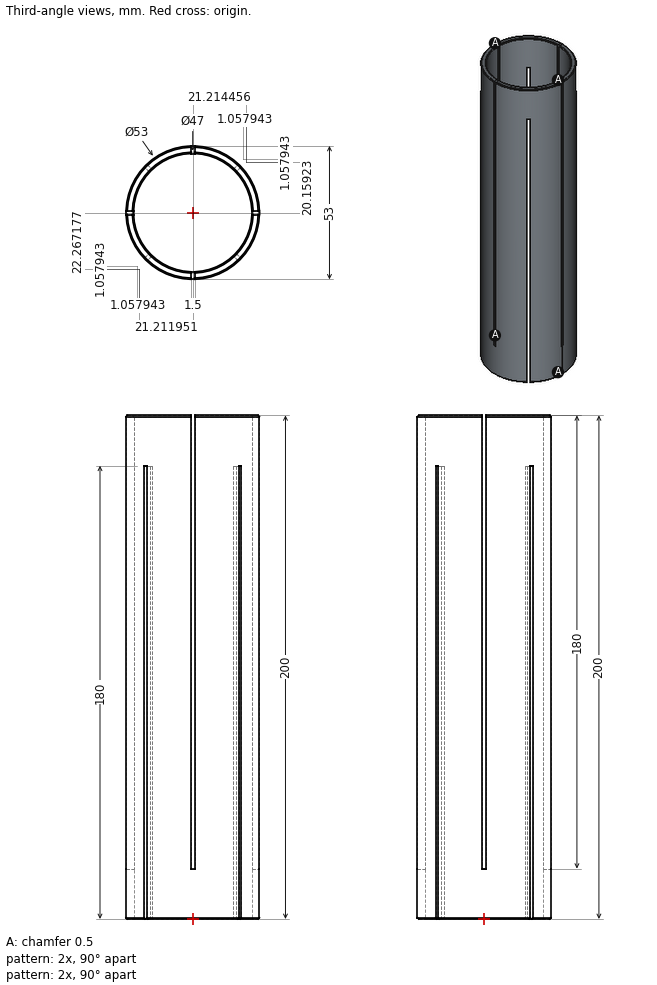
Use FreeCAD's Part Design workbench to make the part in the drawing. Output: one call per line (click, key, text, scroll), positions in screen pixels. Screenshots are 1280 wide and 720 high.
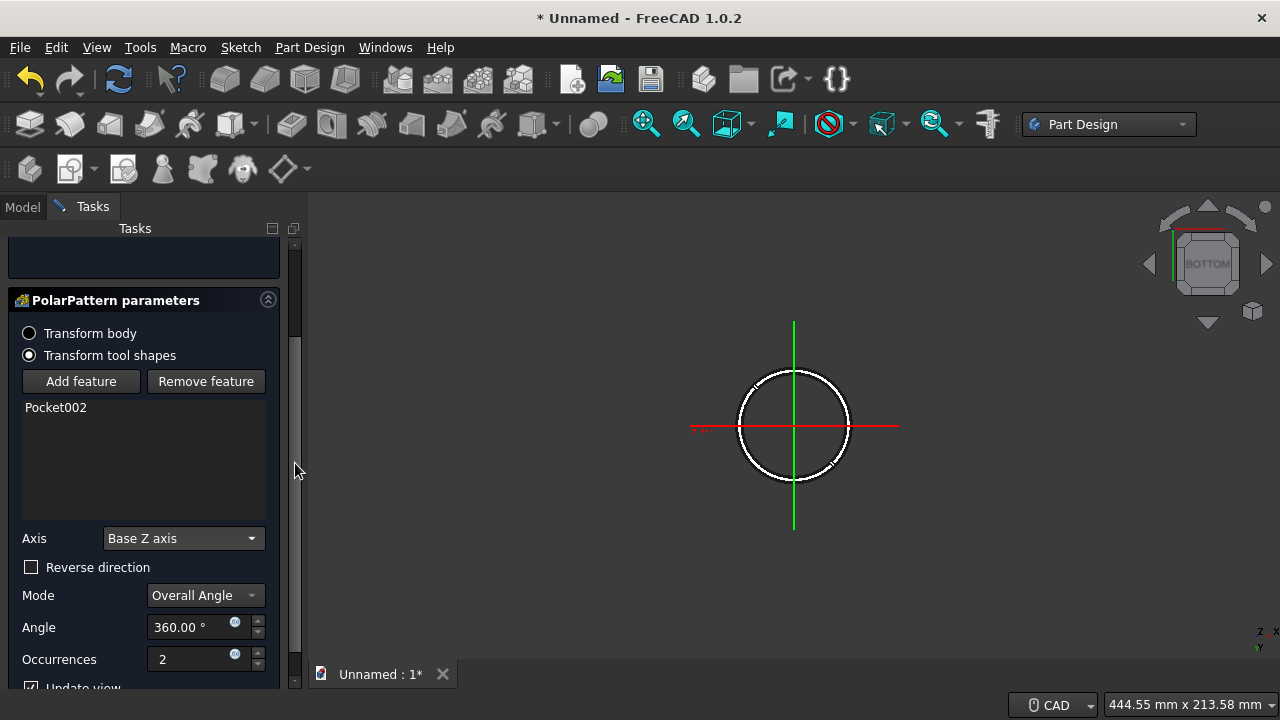
click(206, 596)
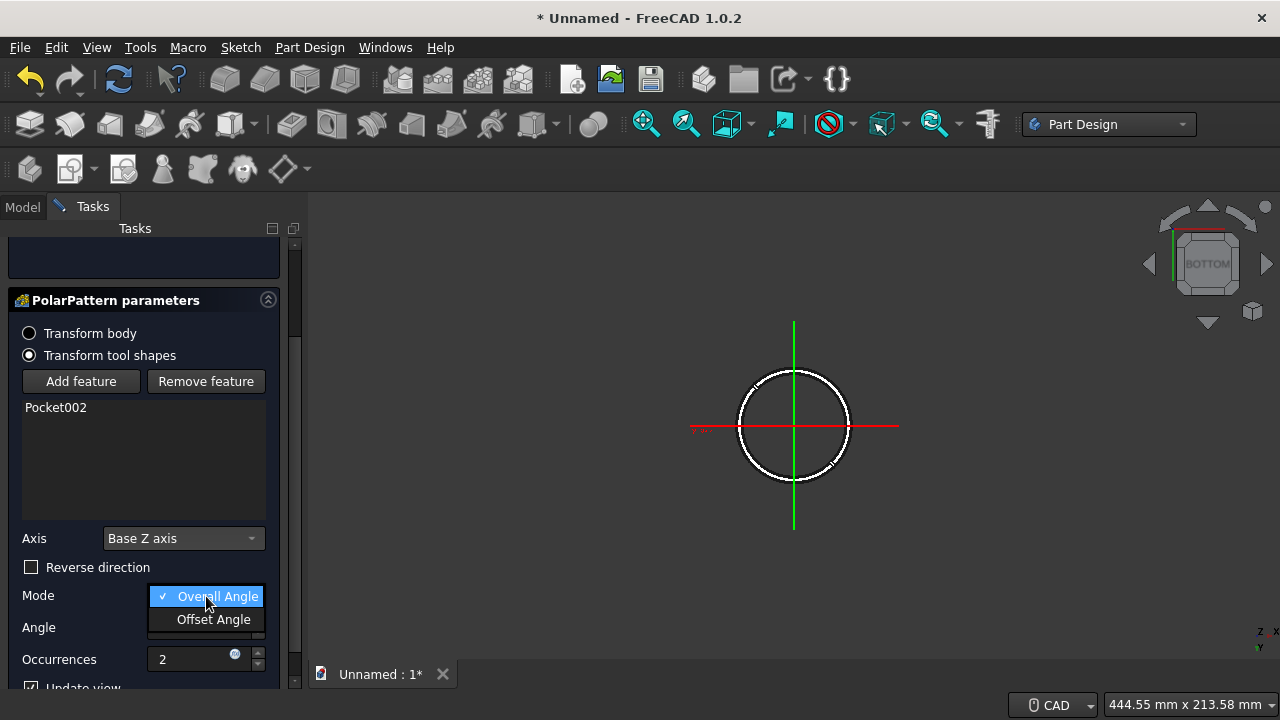
click(206, 620)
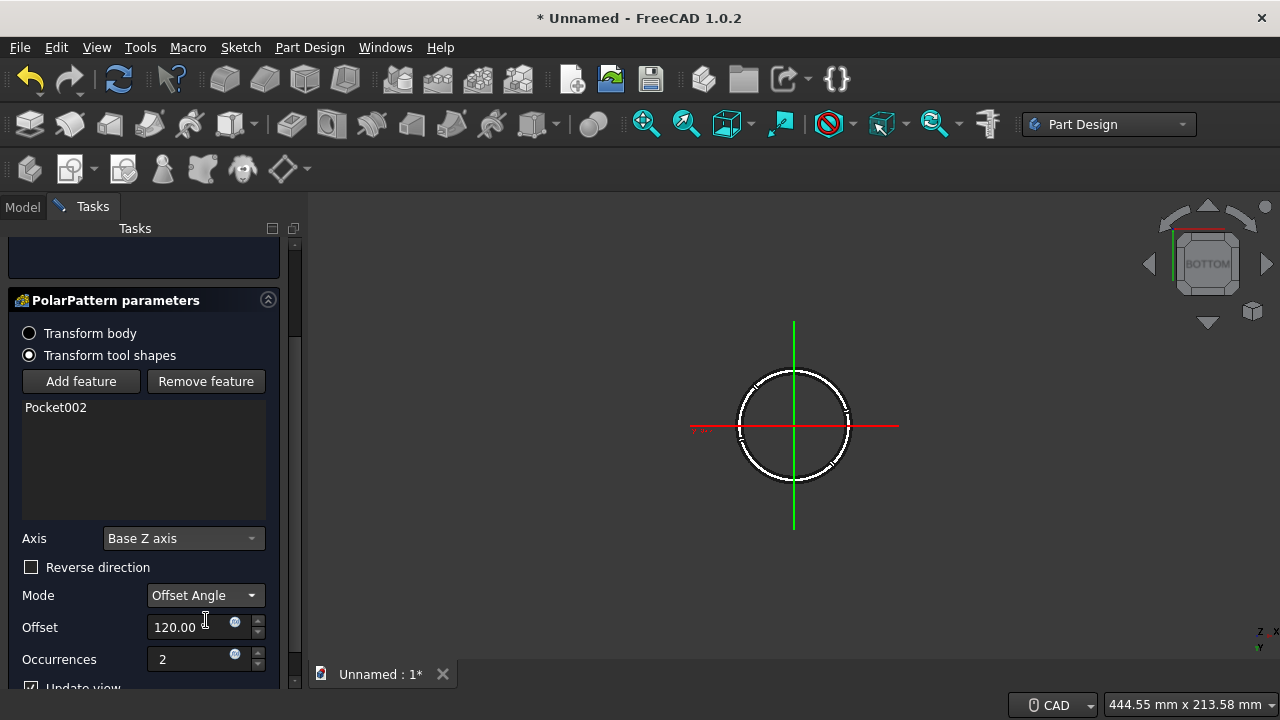
triple_click(198, 627)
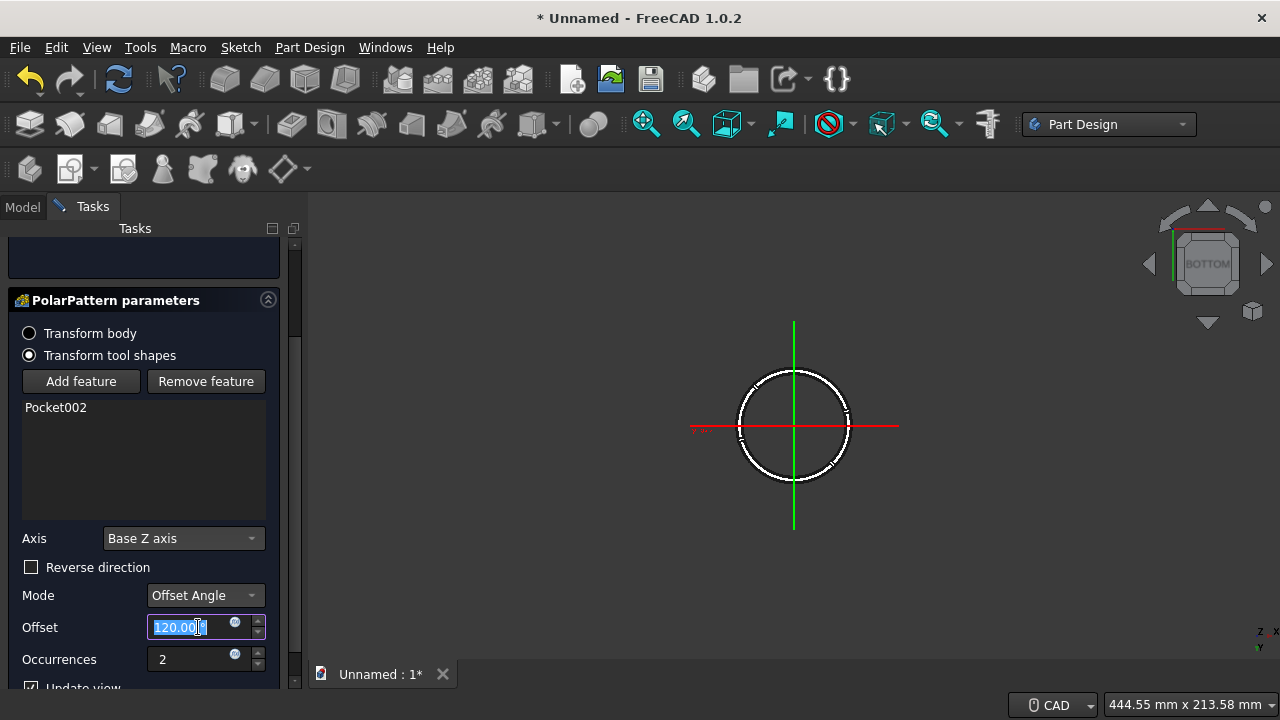
text(90)
key(Tab)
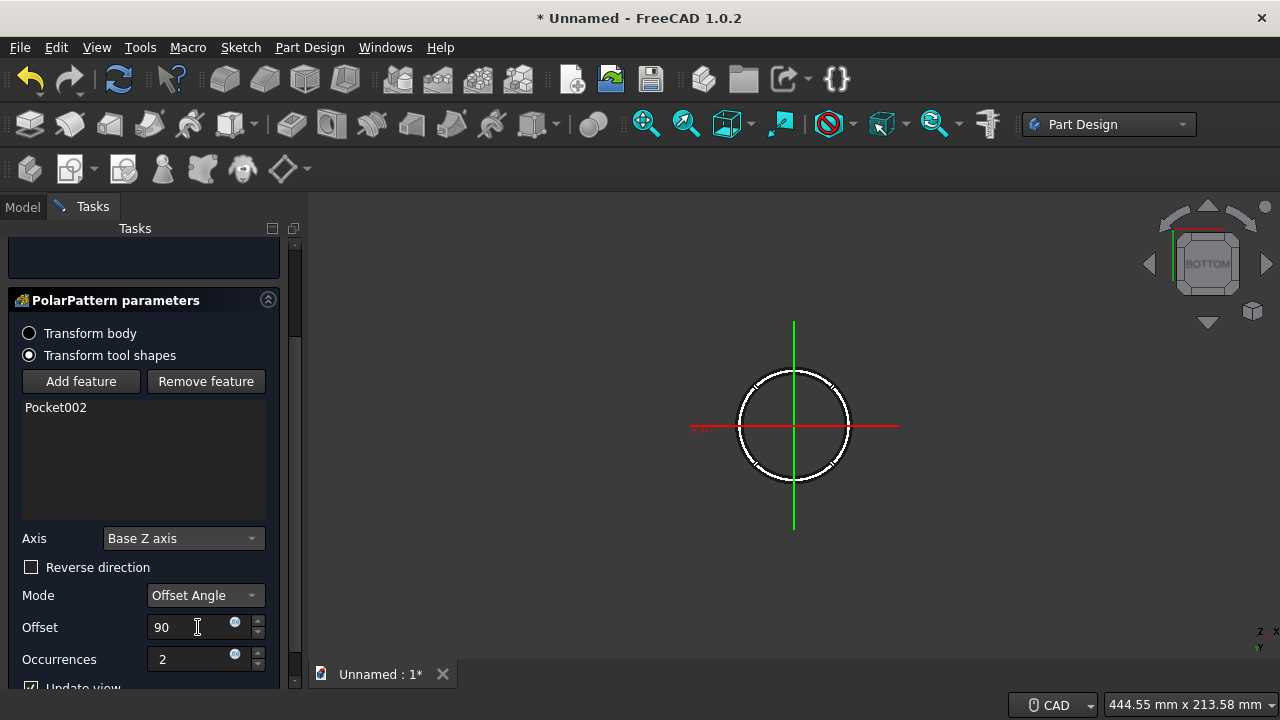
triple_click(198, 659)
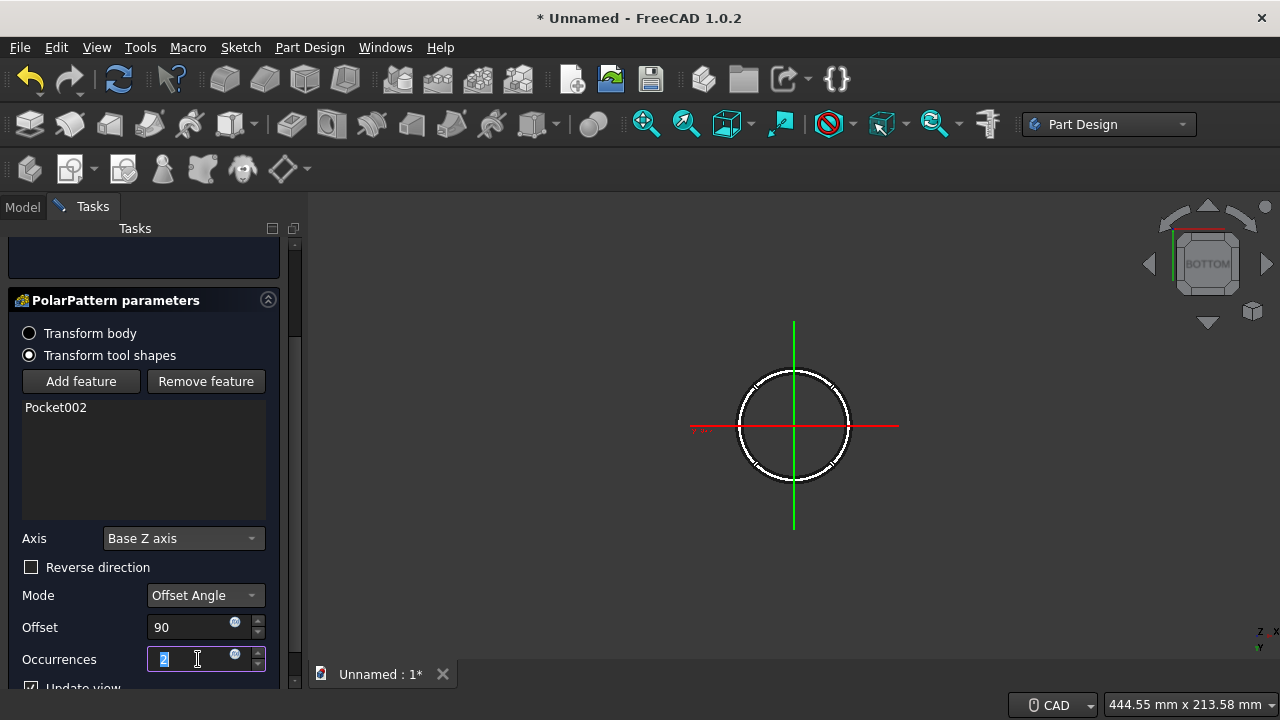
text(2)
key(Tab)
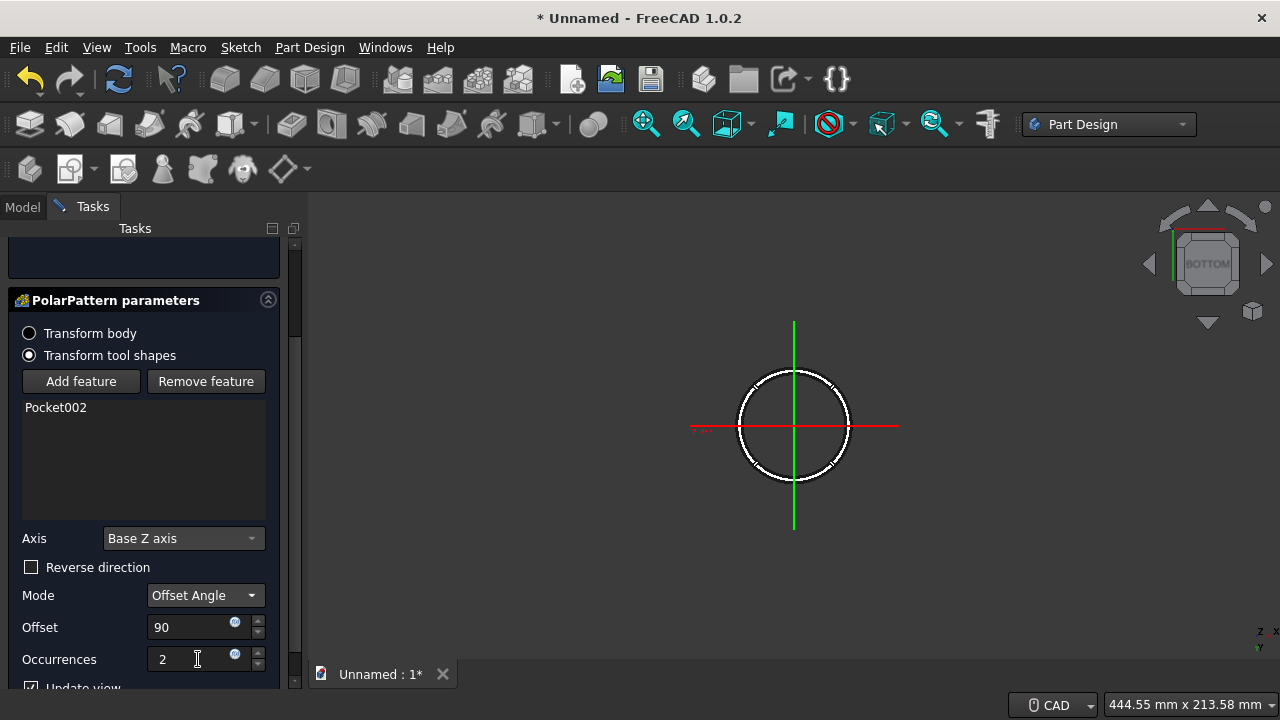
scroll(295, 463, up, 3)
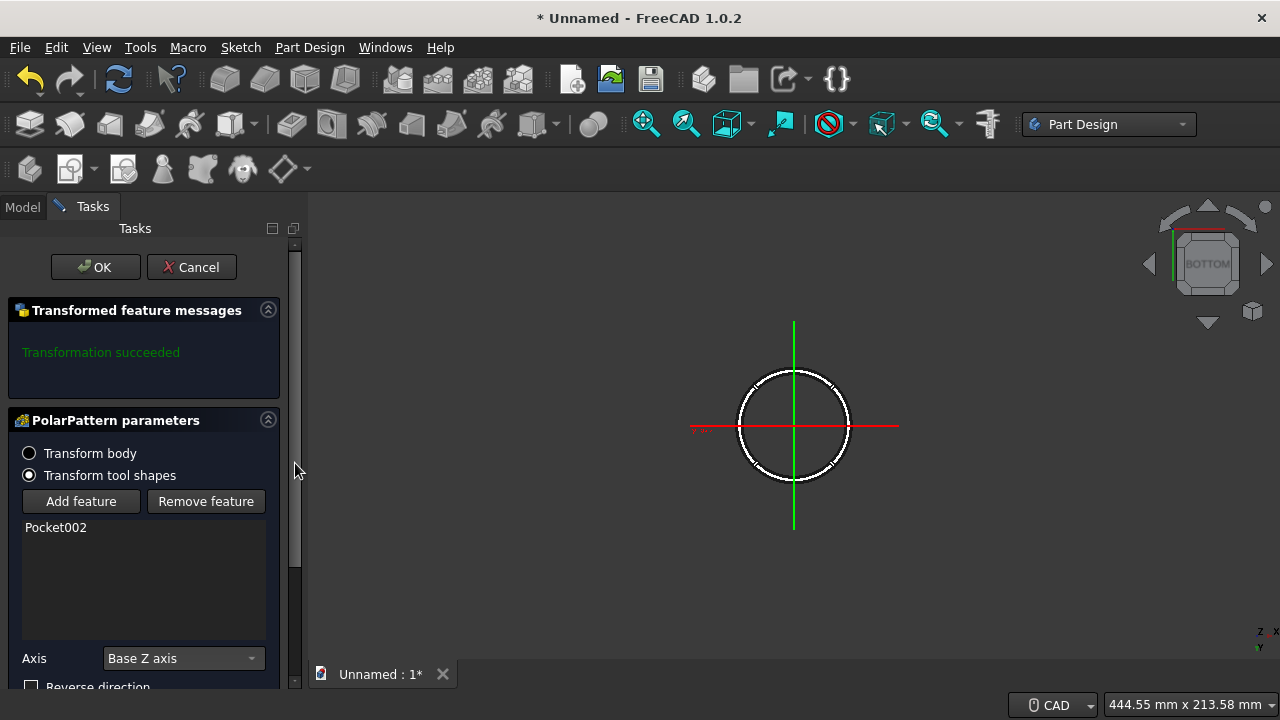
click(96, 267)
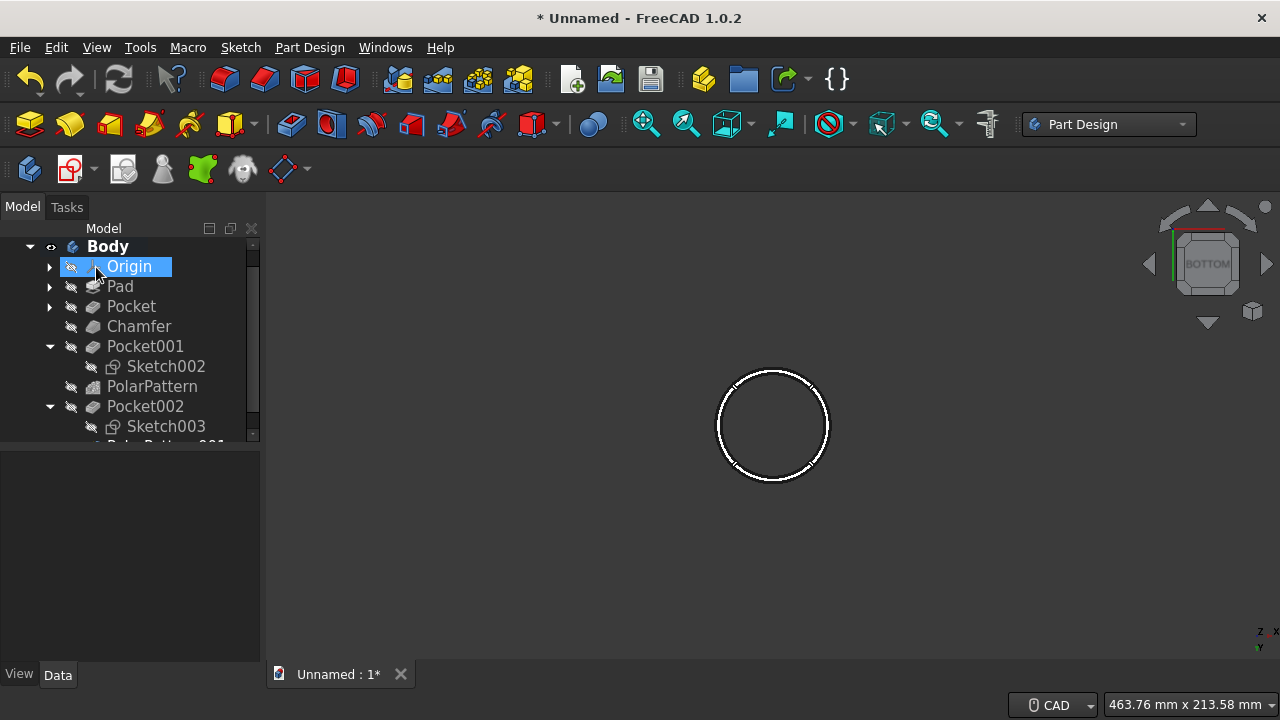
key(0)